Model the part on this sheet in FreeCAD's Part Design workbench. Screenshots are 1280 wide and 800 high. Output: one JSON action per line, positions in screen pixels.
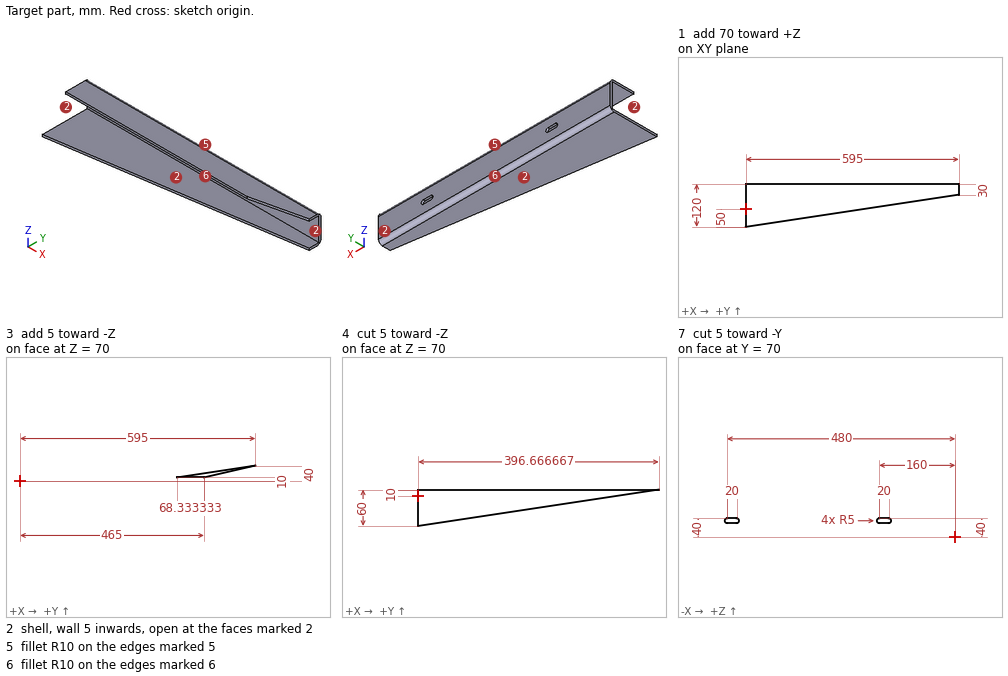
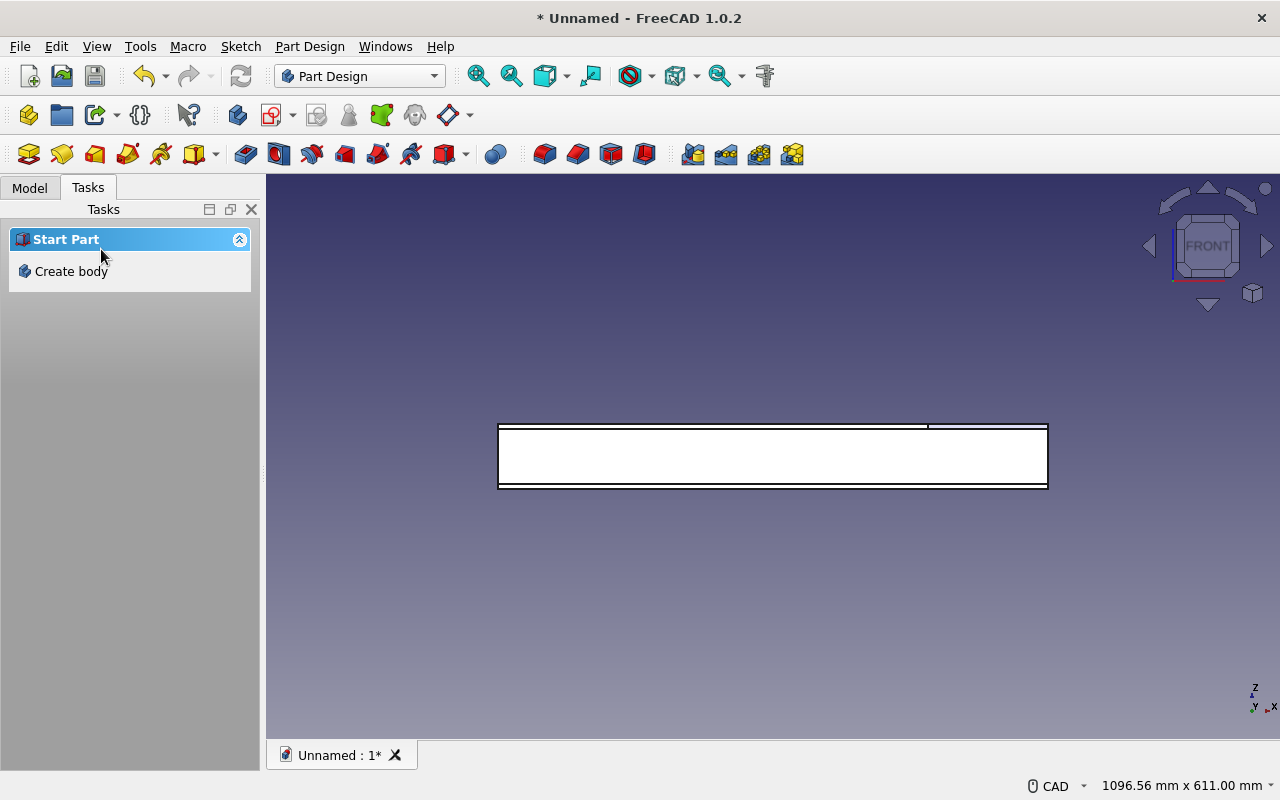
{"action": "key", "text": "3"}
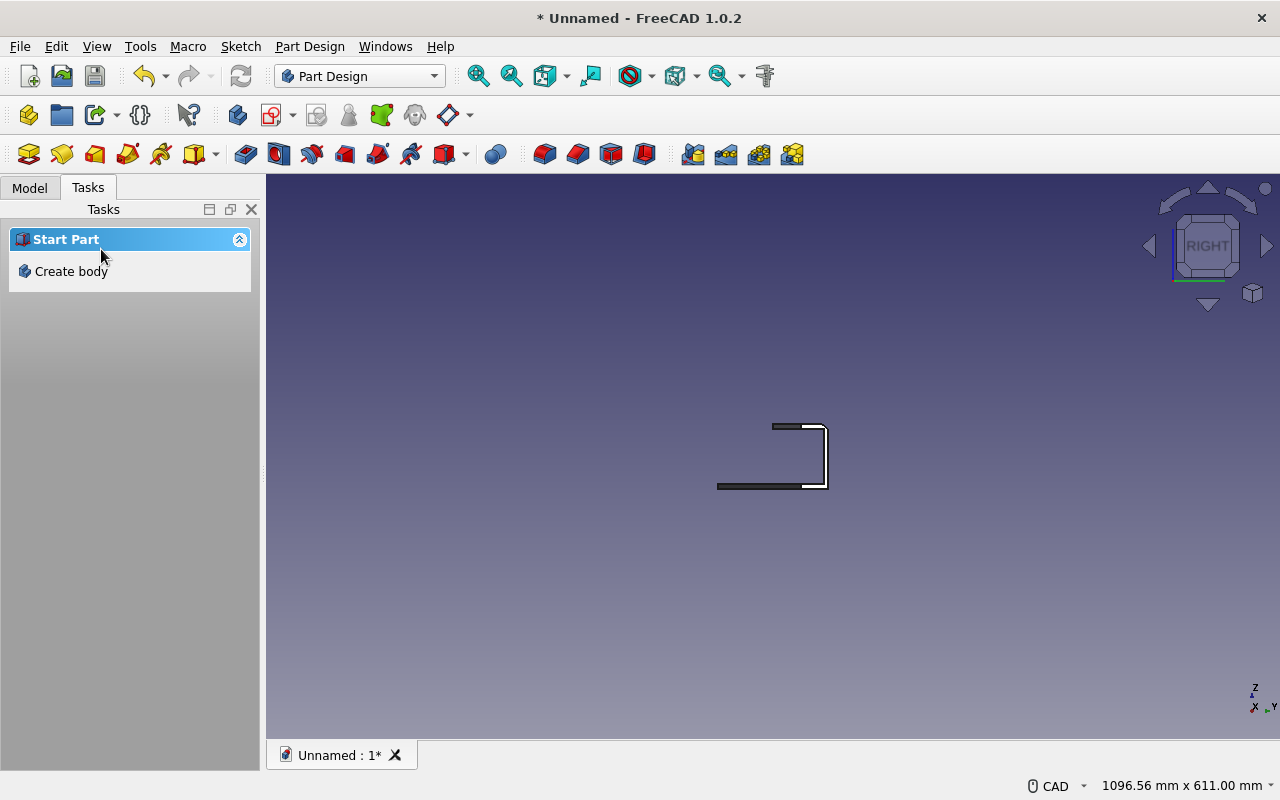
{"action": "left_click", "coordinate": [479, 76]}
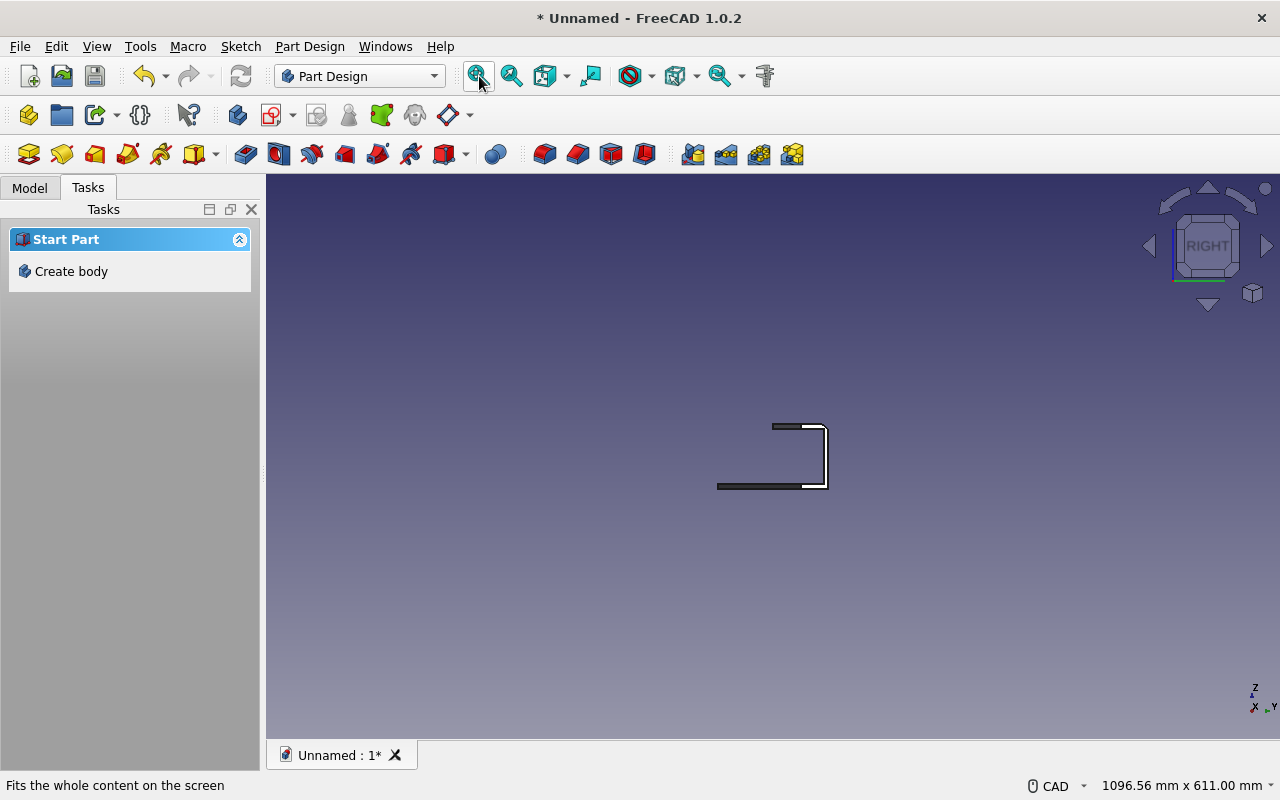
{"action": "key", "text": "5"}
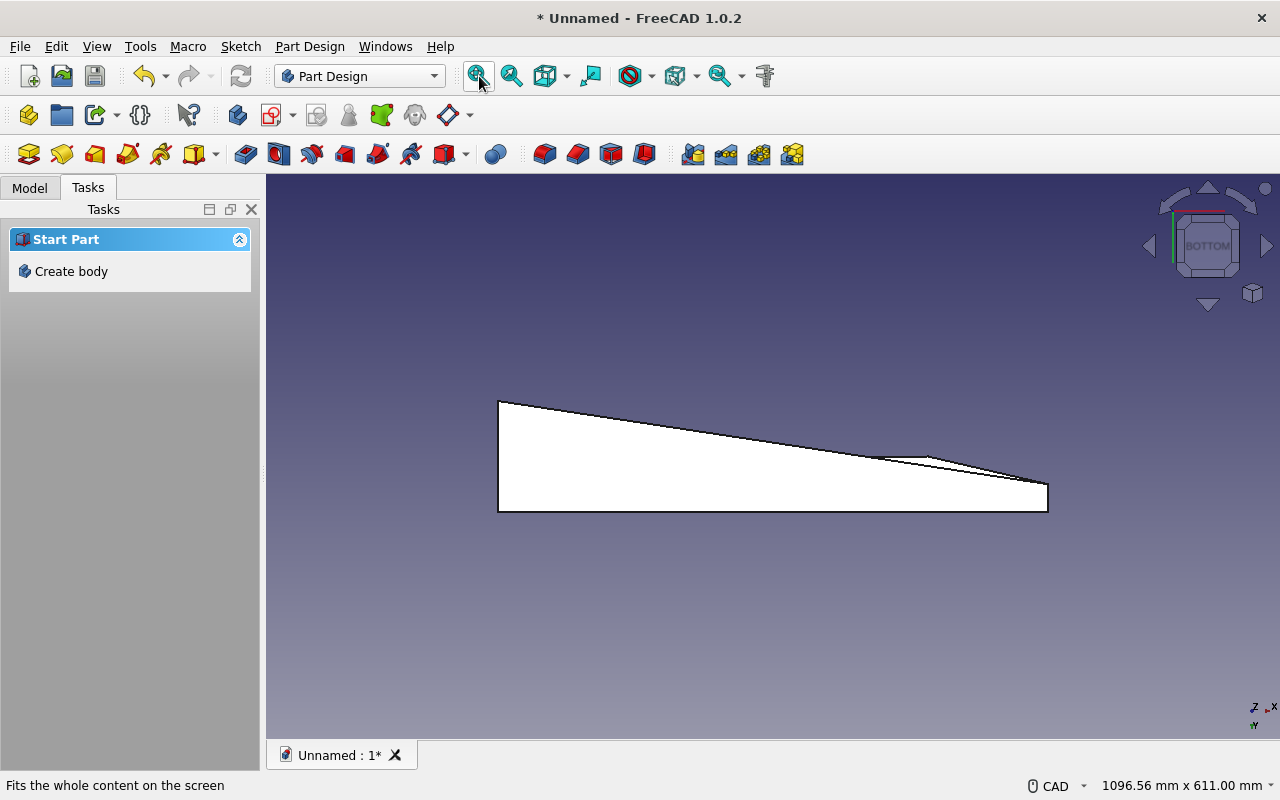
{"action": "left_click", "coordinate": [773, 511]}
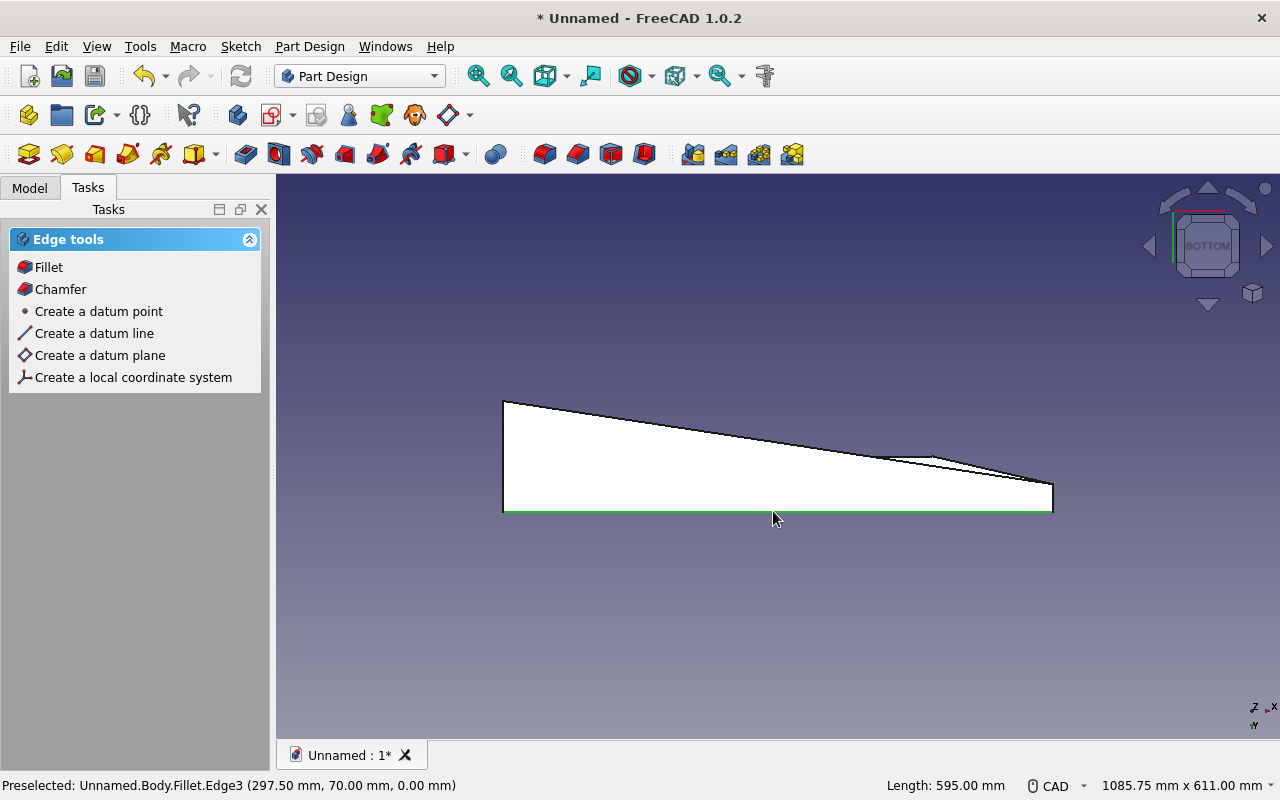
{"action": "left_click", "coordinate": [545, 154]}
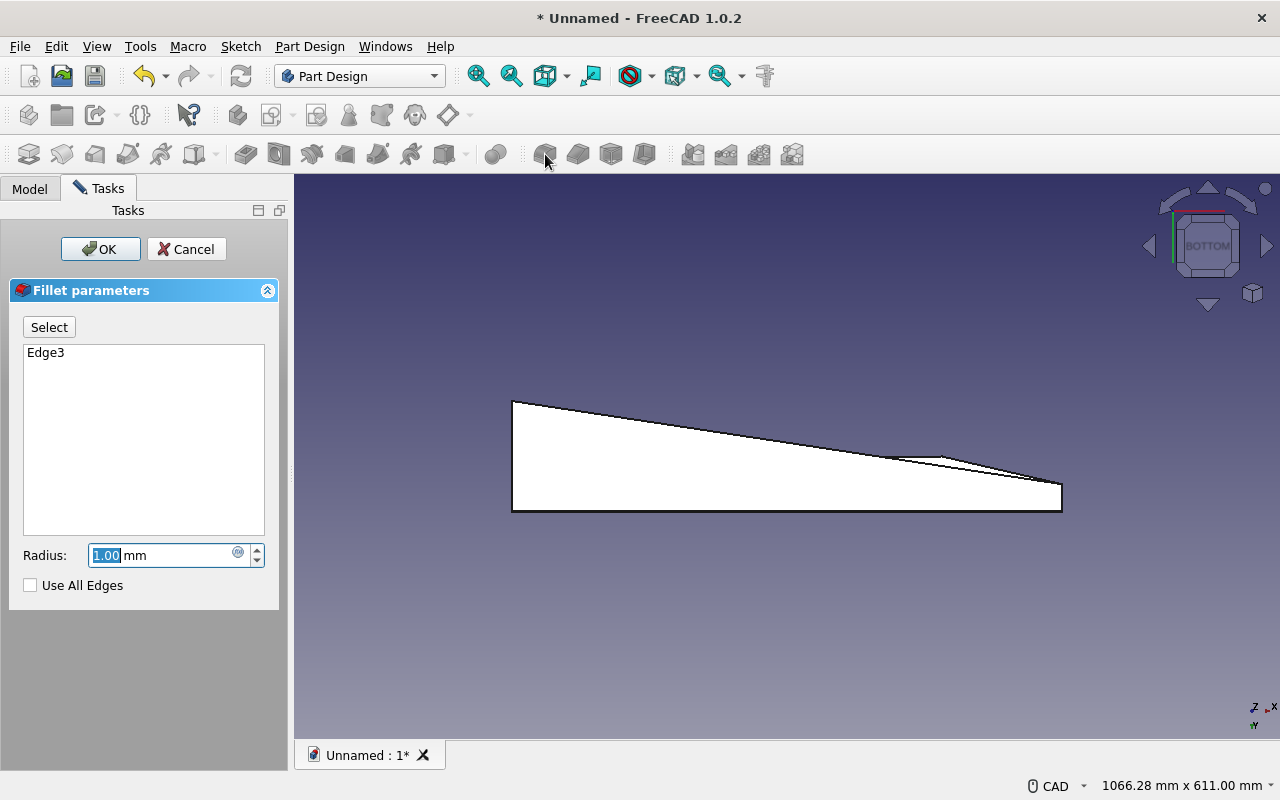
{"action": "type", "text": "10"}
{"action": "key", "text": "Tab"}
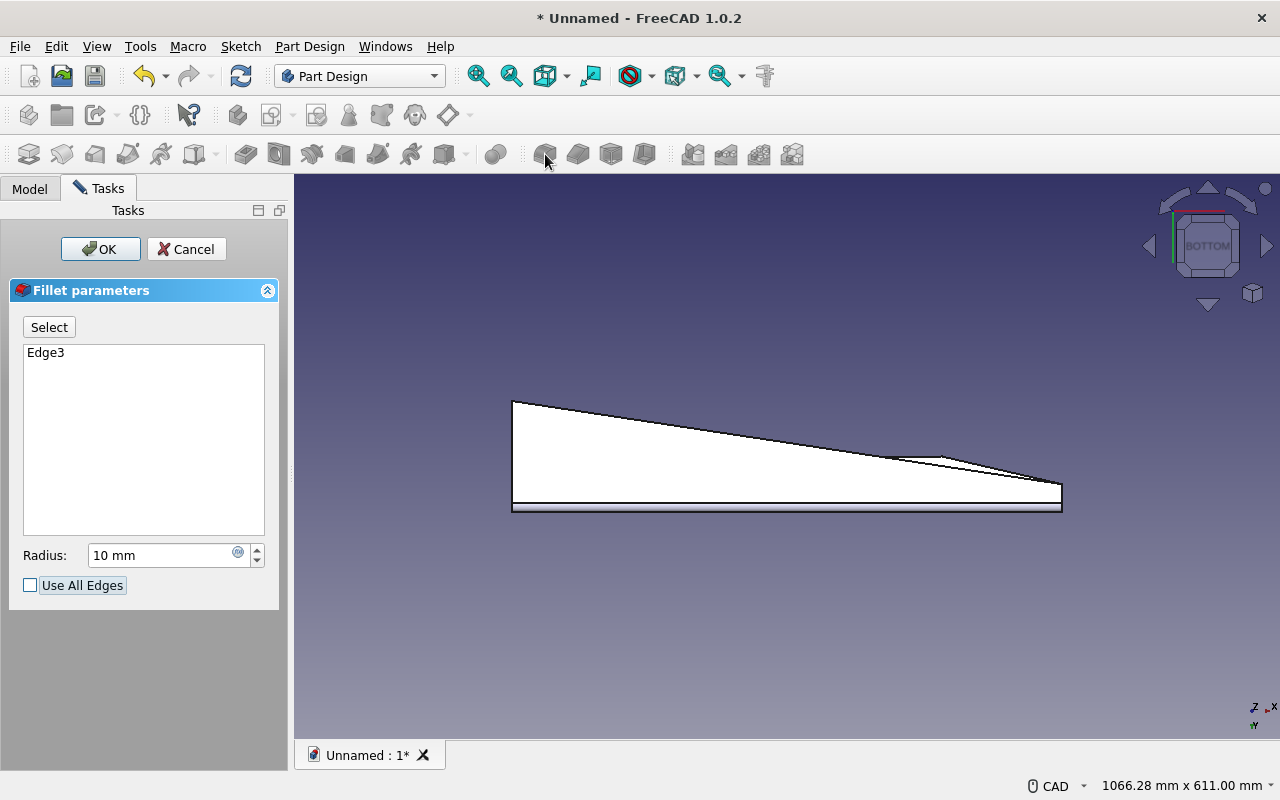
{"action": "left_click", "coordinate": [101, 249]}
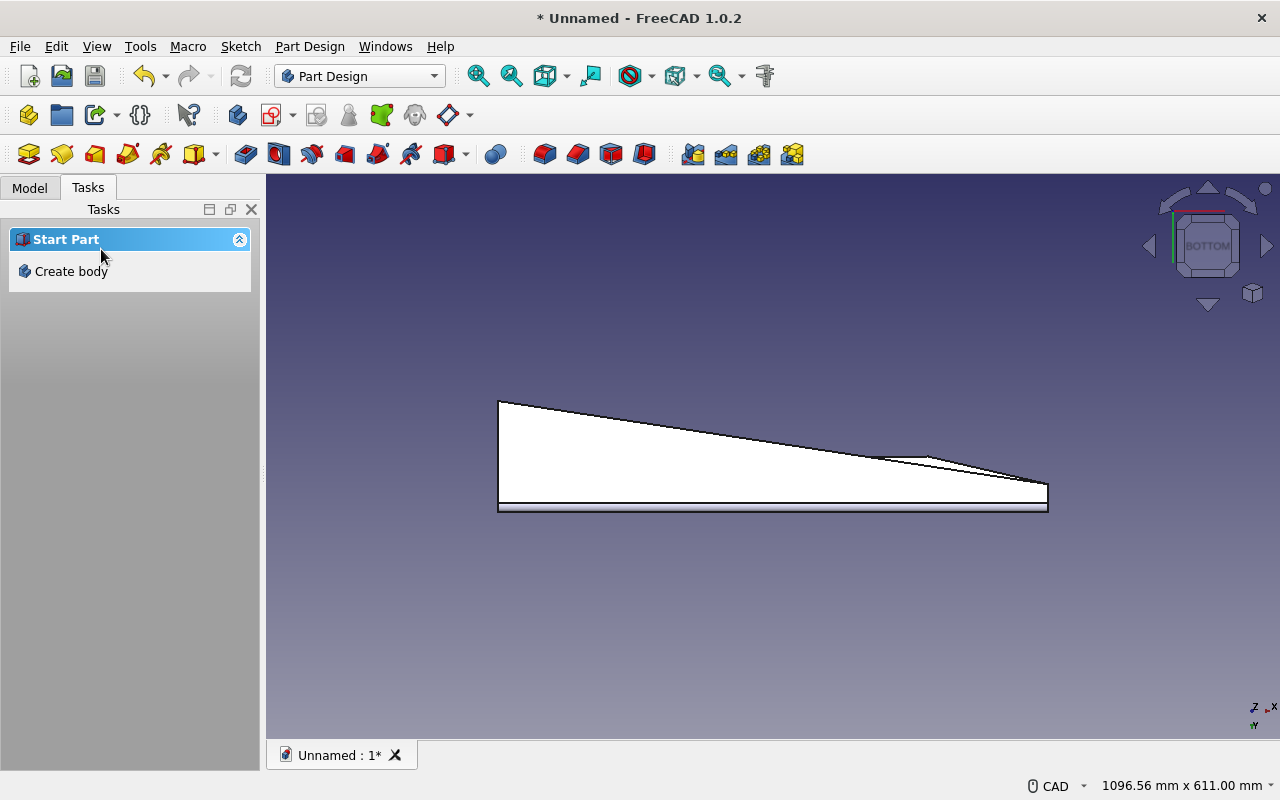
{"action": "key", "text": "4"}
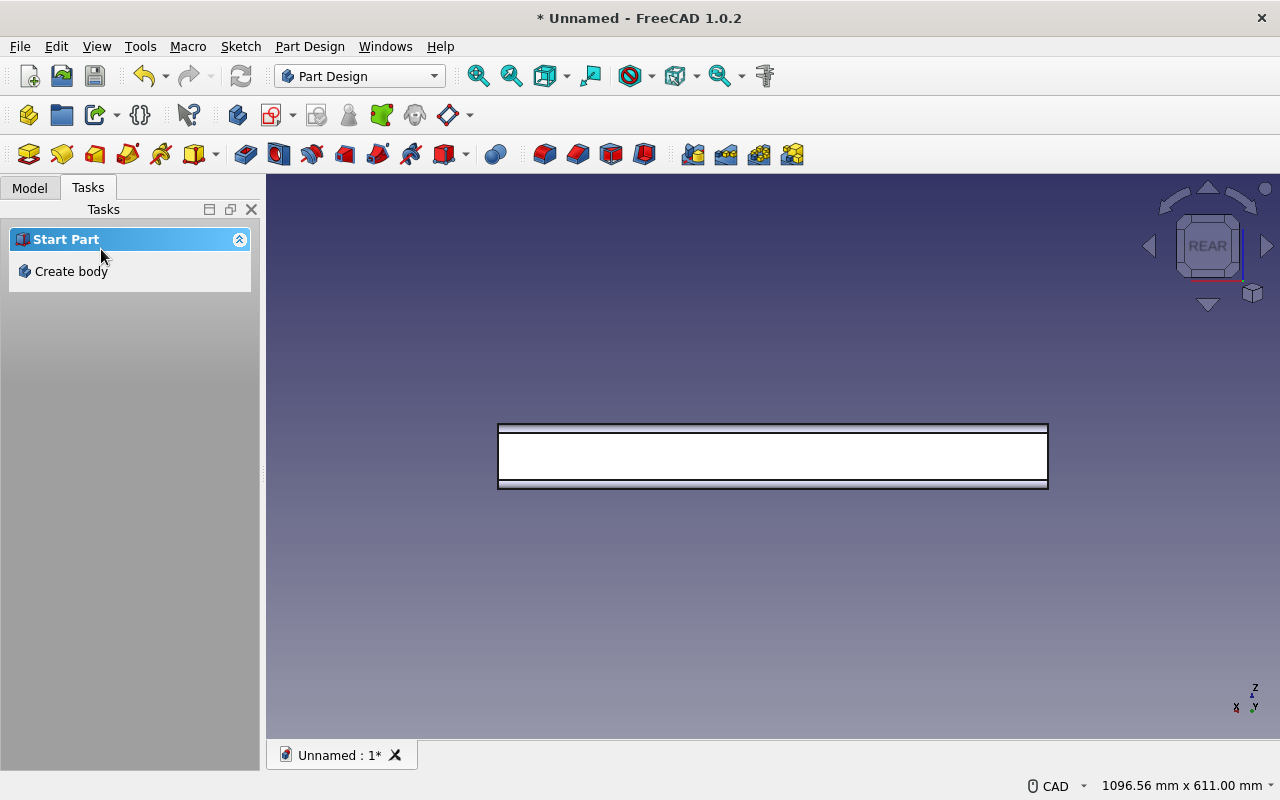
{"action": "left_click", "coordinate": [537, 456]}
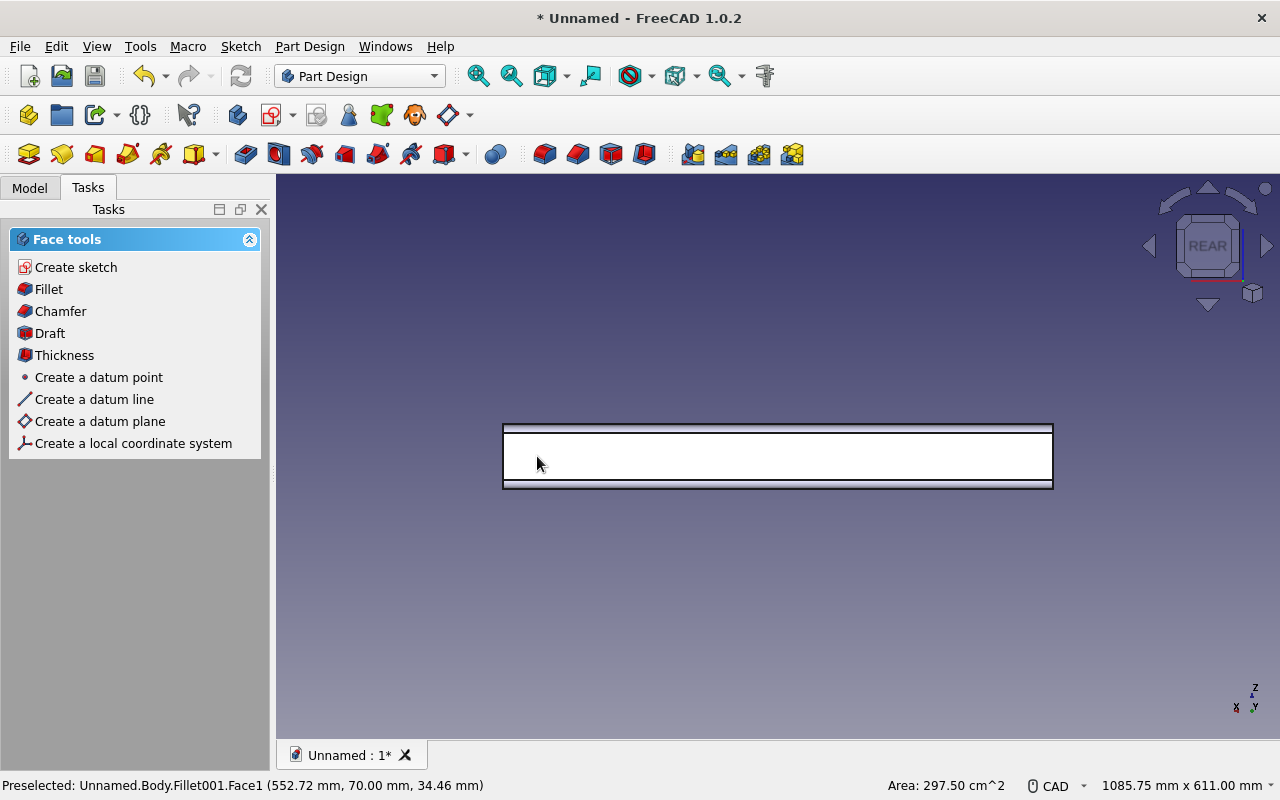
{"action": "left_click", "coordinate": [270, 116]}